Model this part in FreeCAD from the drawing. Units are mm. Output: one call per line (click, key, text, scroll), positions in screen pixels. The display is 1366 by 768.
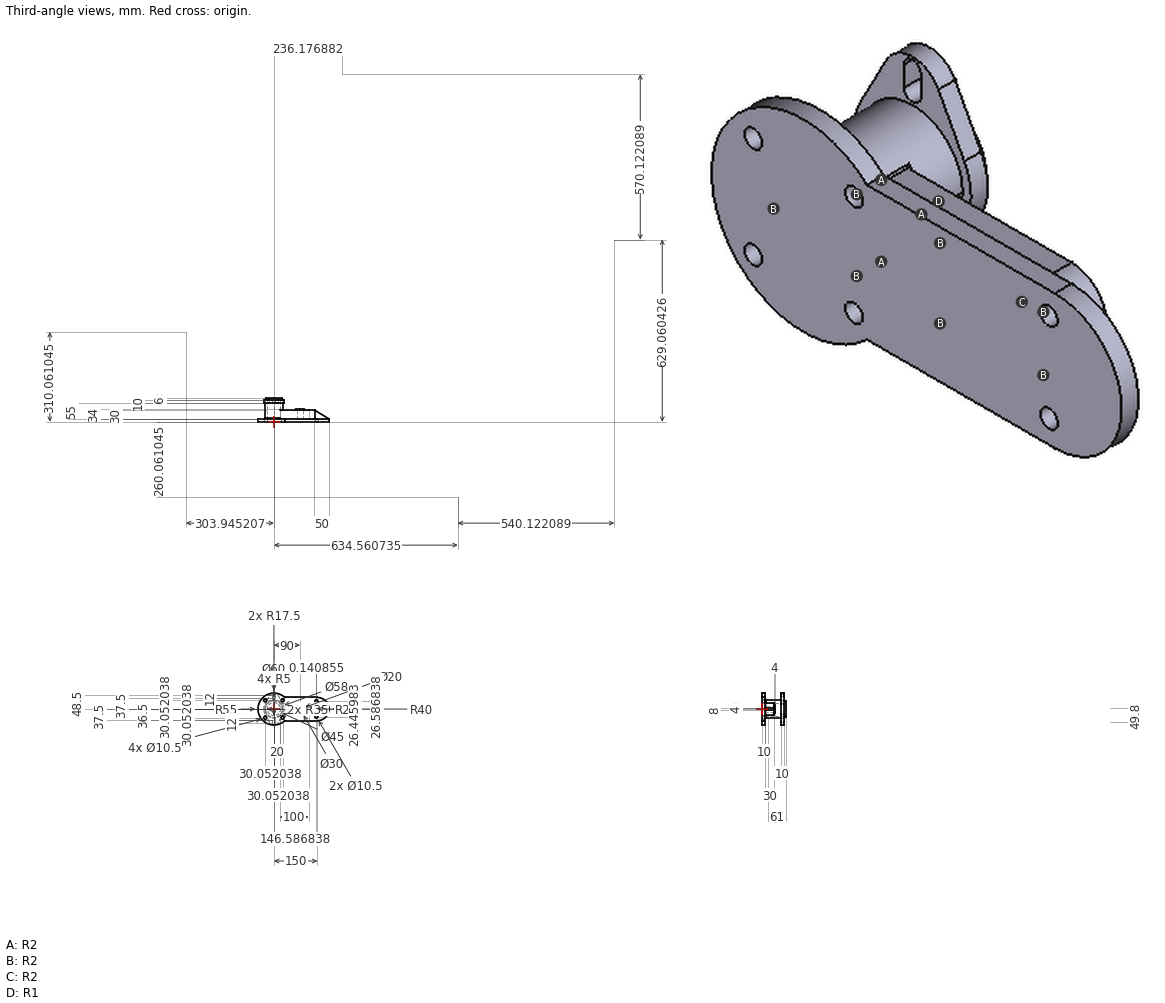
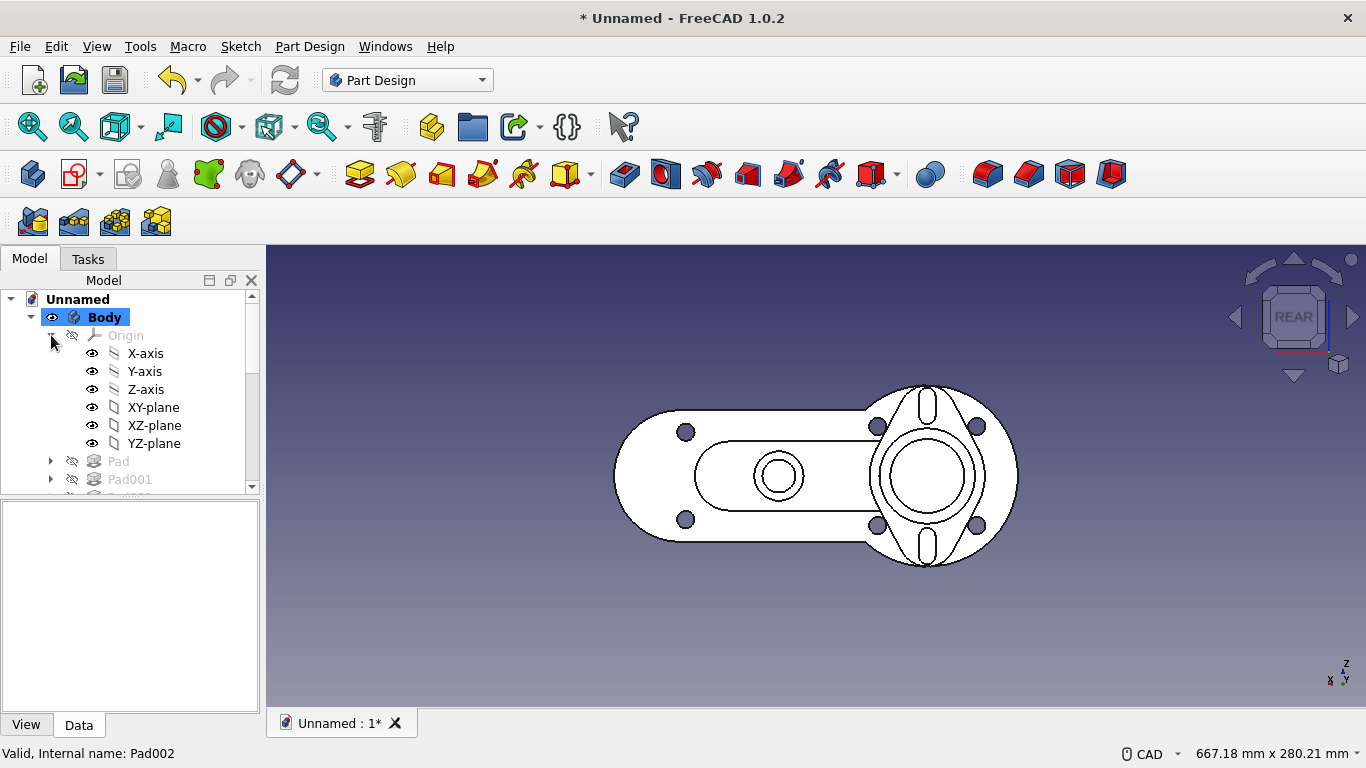
click(137, 443)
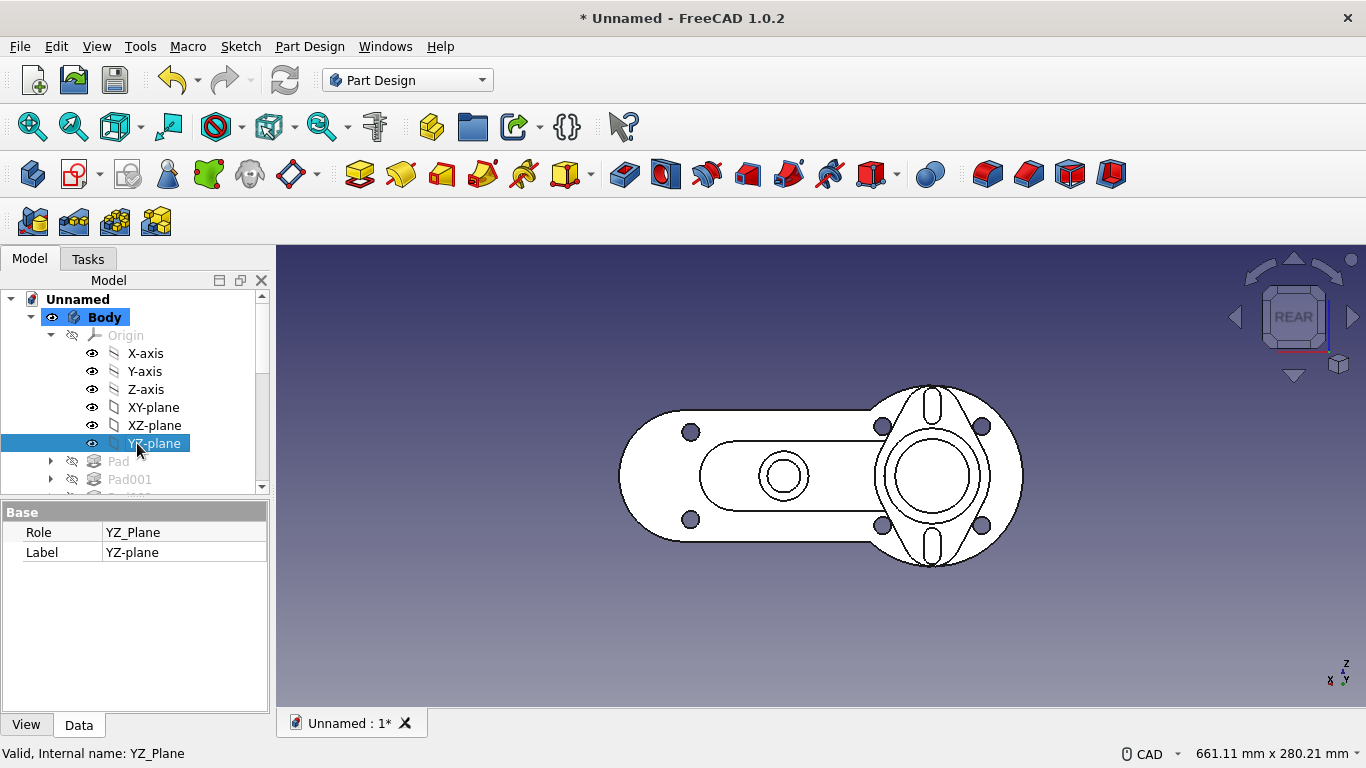
click(290, 174)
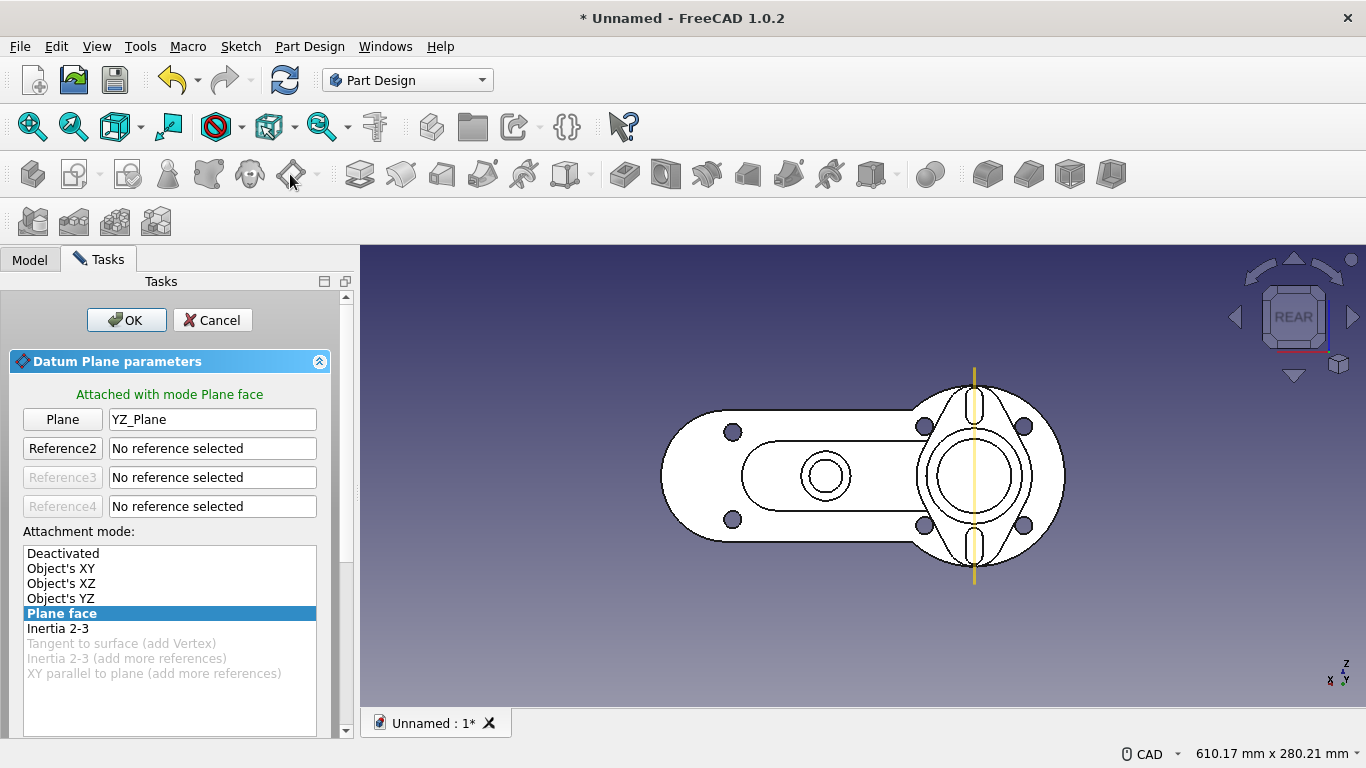
scroll(346, 514, down, 4)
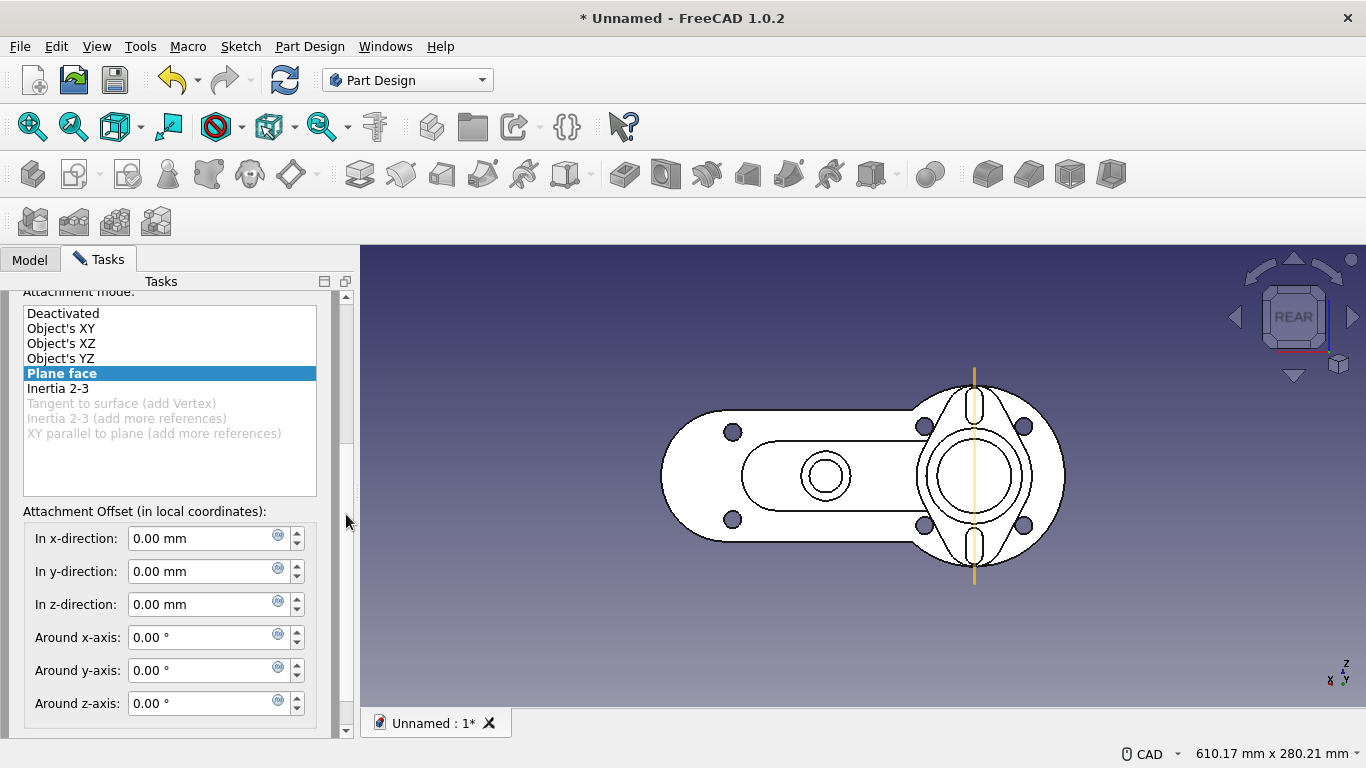
triple_click(210, 604)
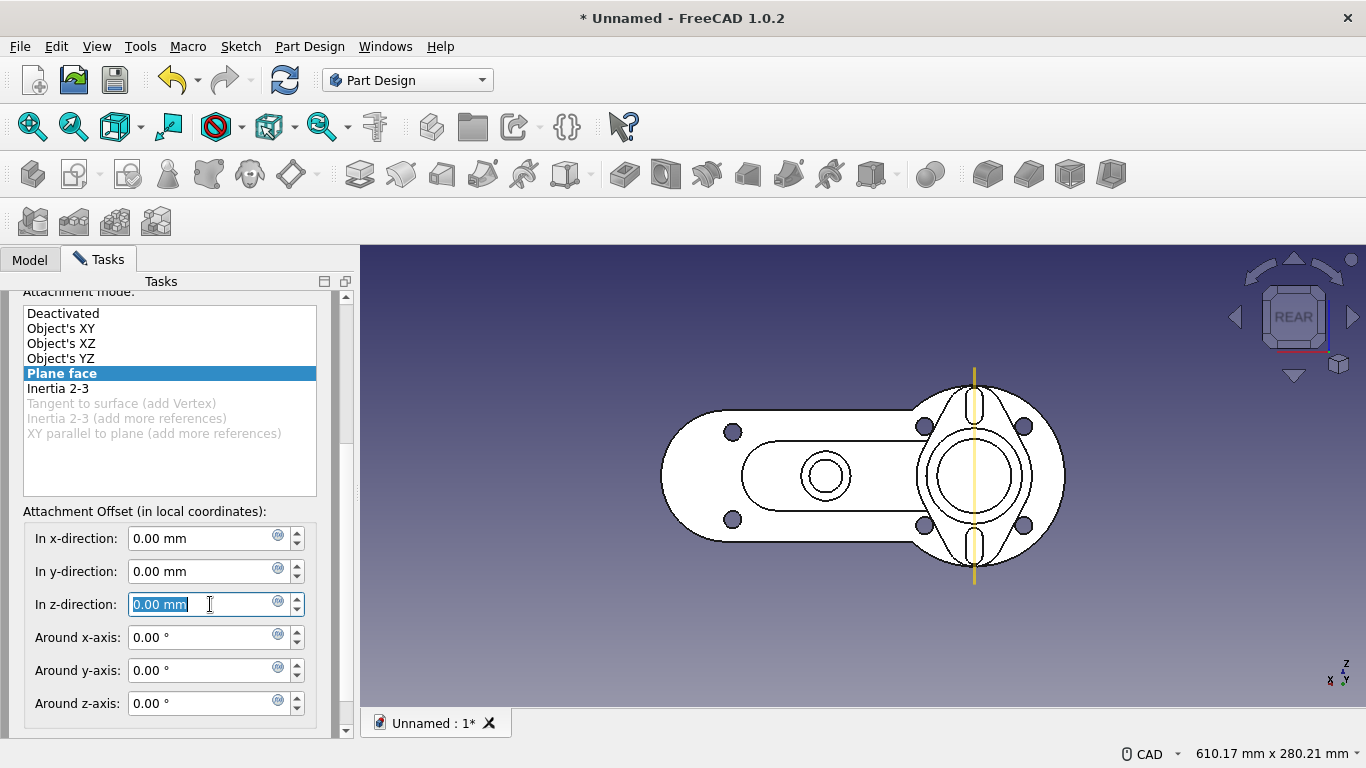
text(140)
key(Tab)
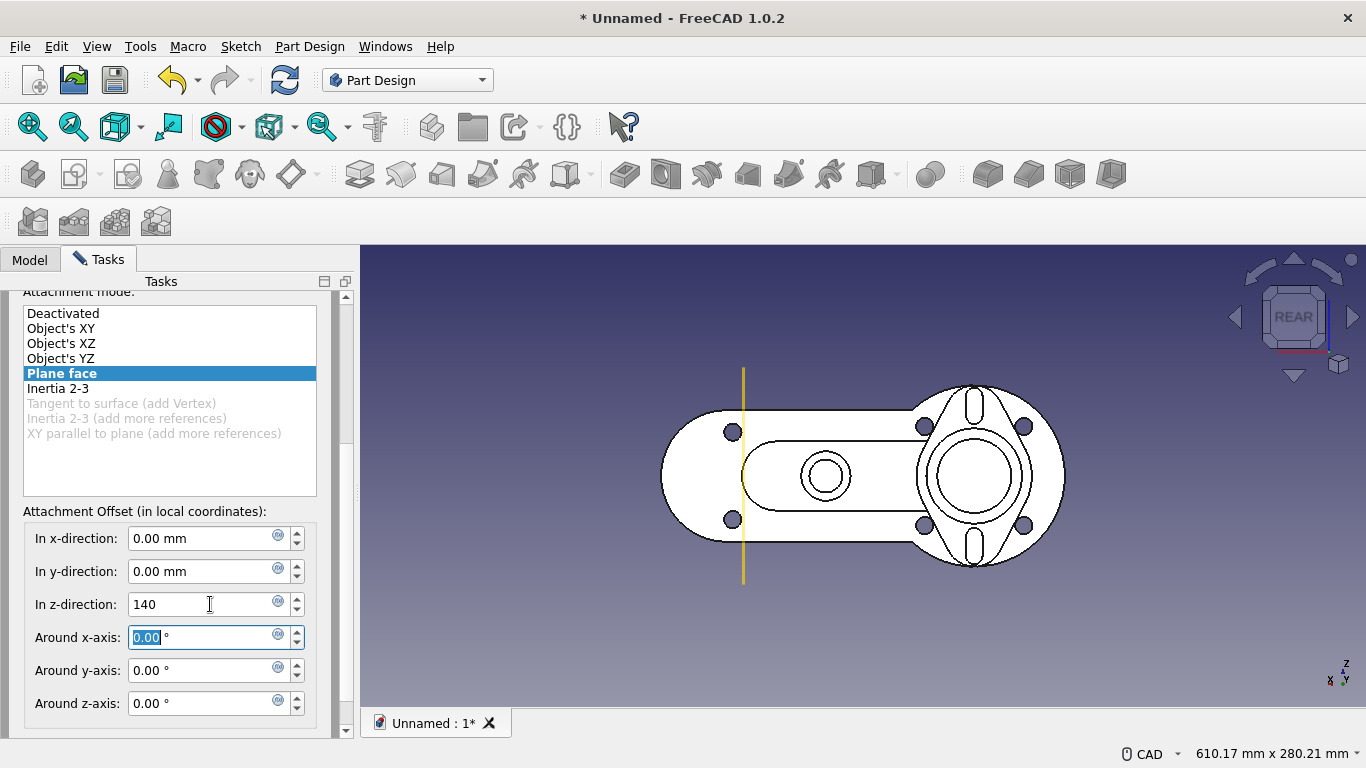
scroll(346, 514, up, 5)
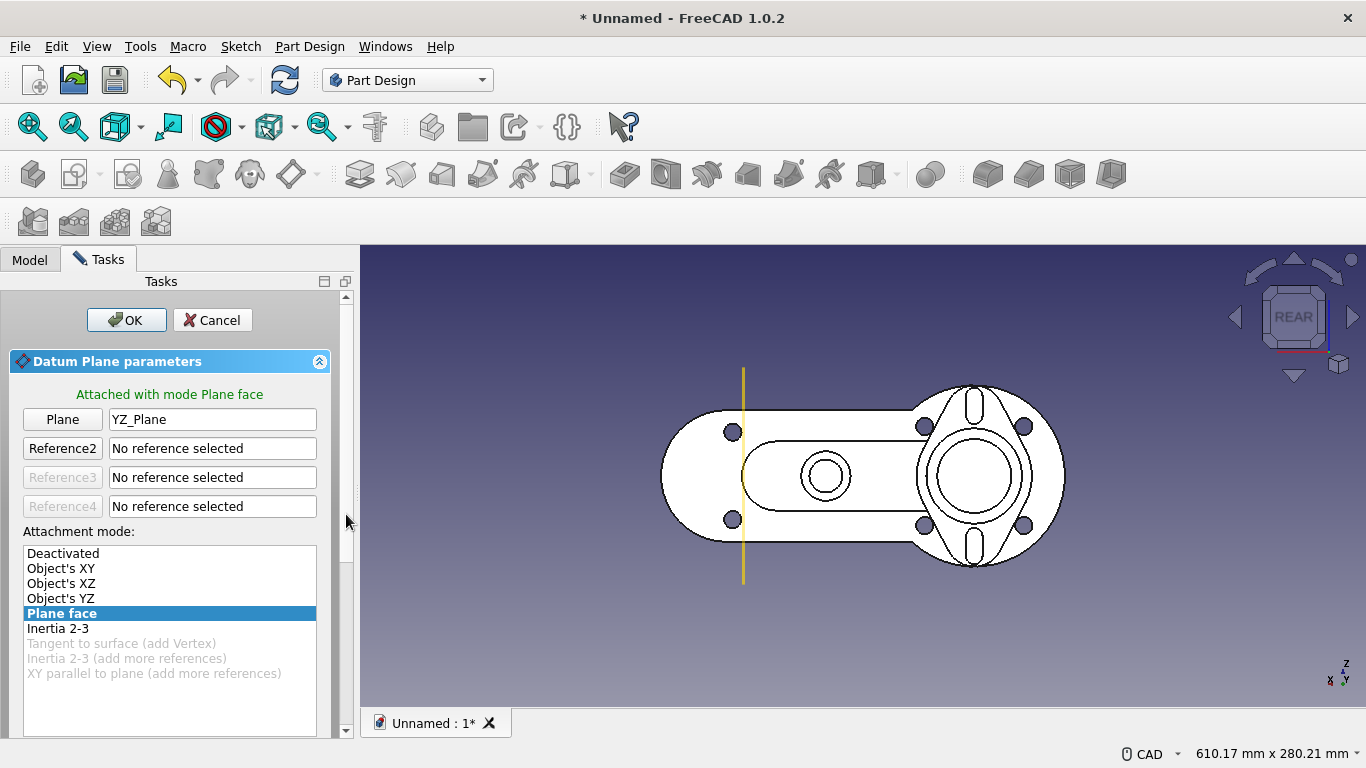
click(127, 320)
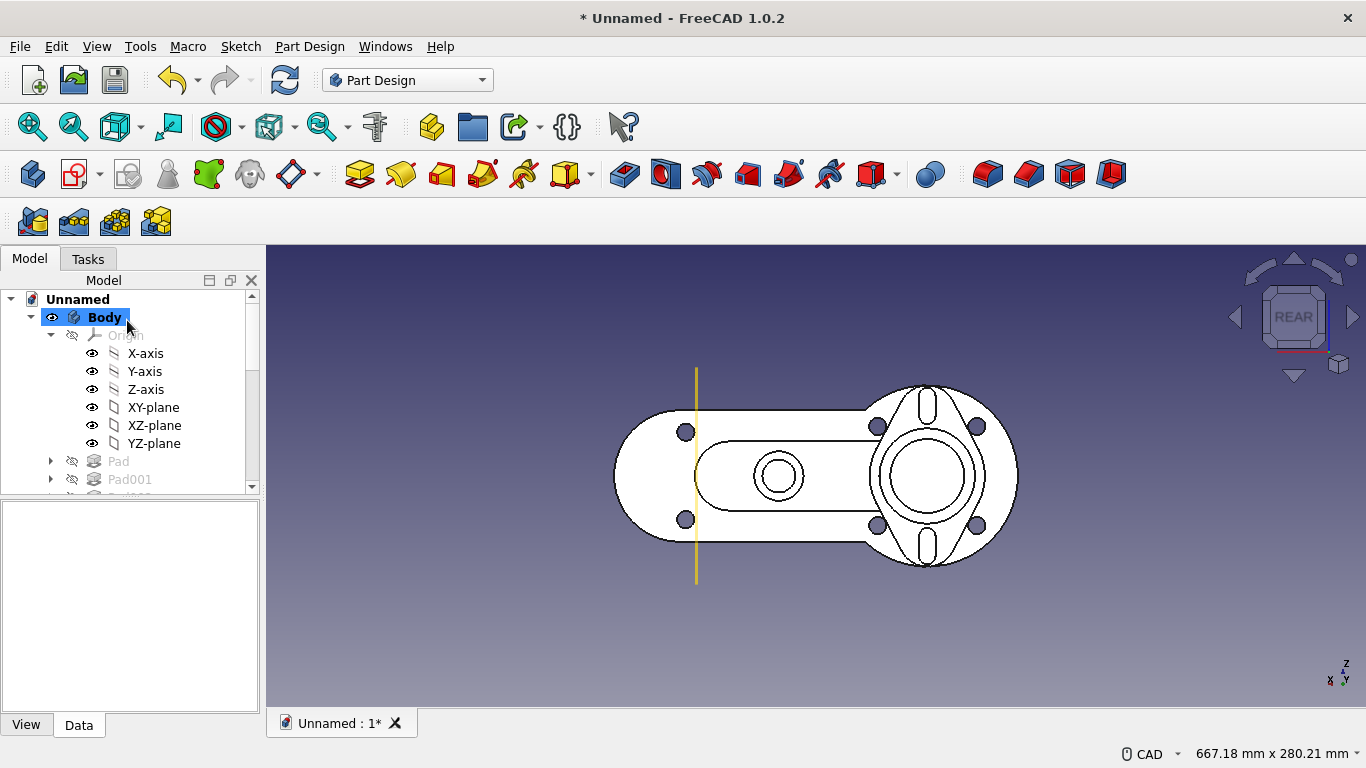
scroll(101, 385, down, 3)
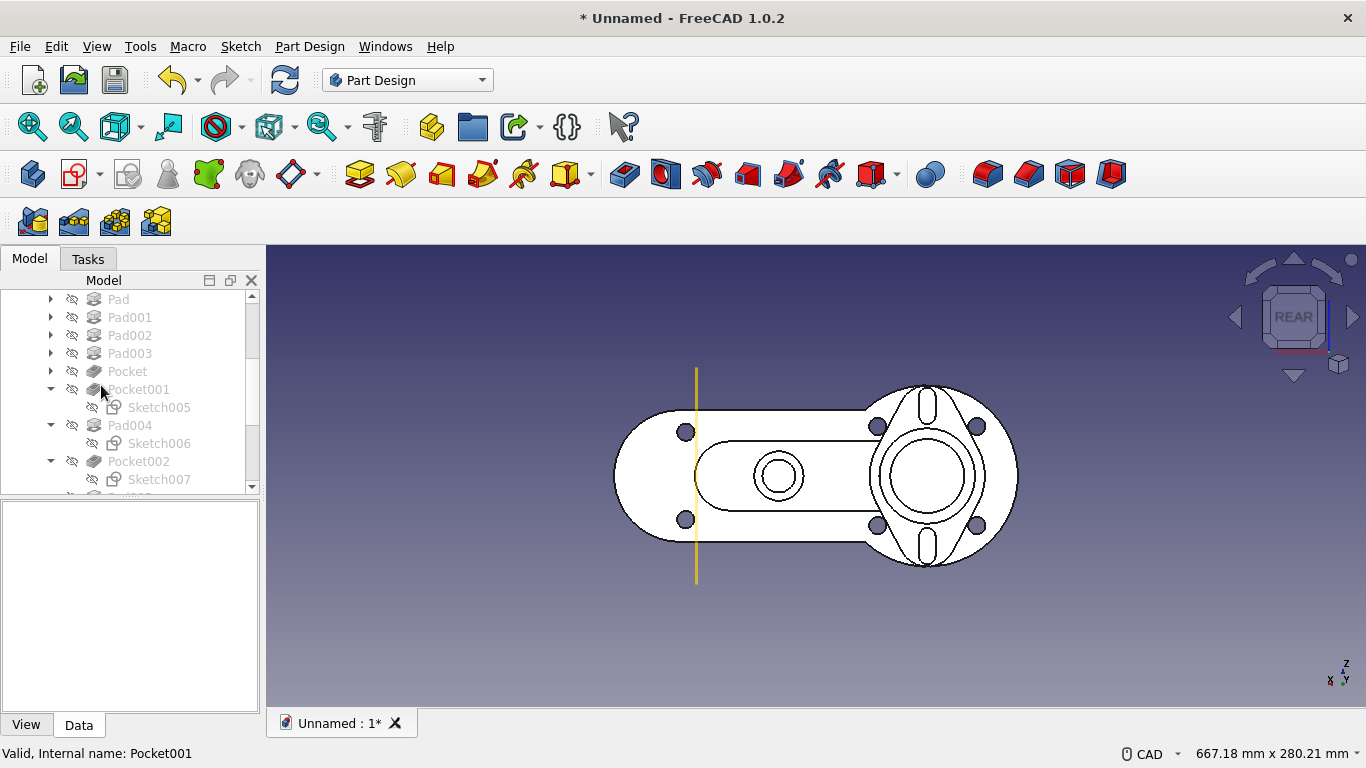
scroll(141, 385, up, 15)